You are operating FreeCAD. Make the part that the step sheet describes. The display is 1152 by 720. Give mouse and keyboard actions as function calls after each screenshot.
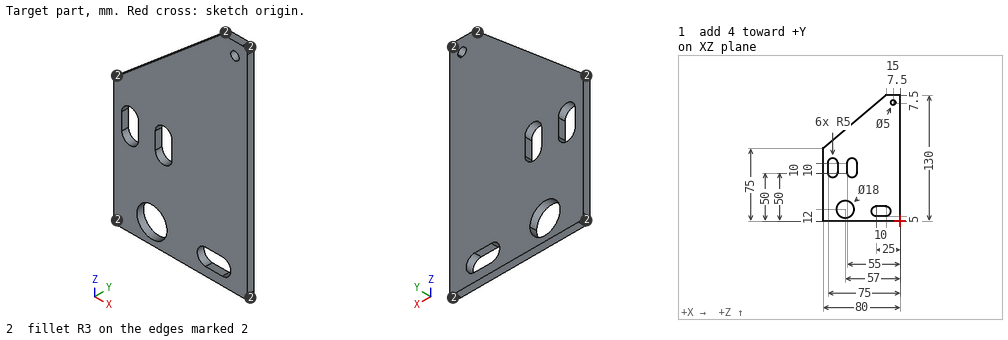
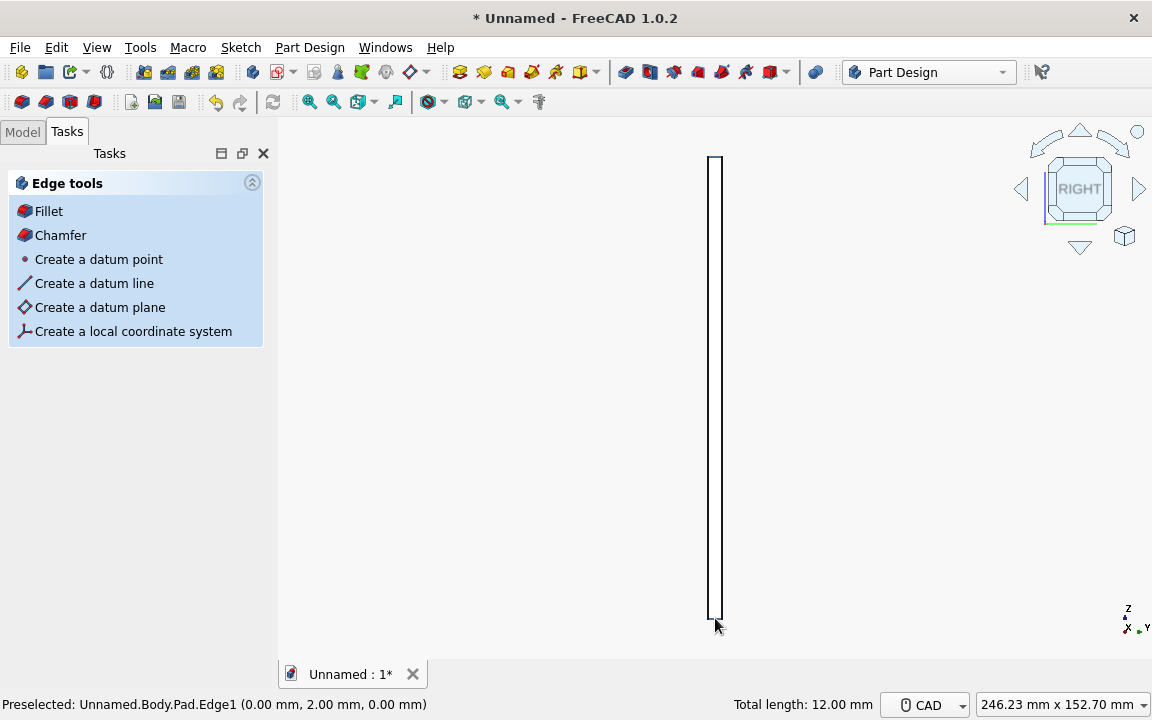
scroll(715, 352, up, 6)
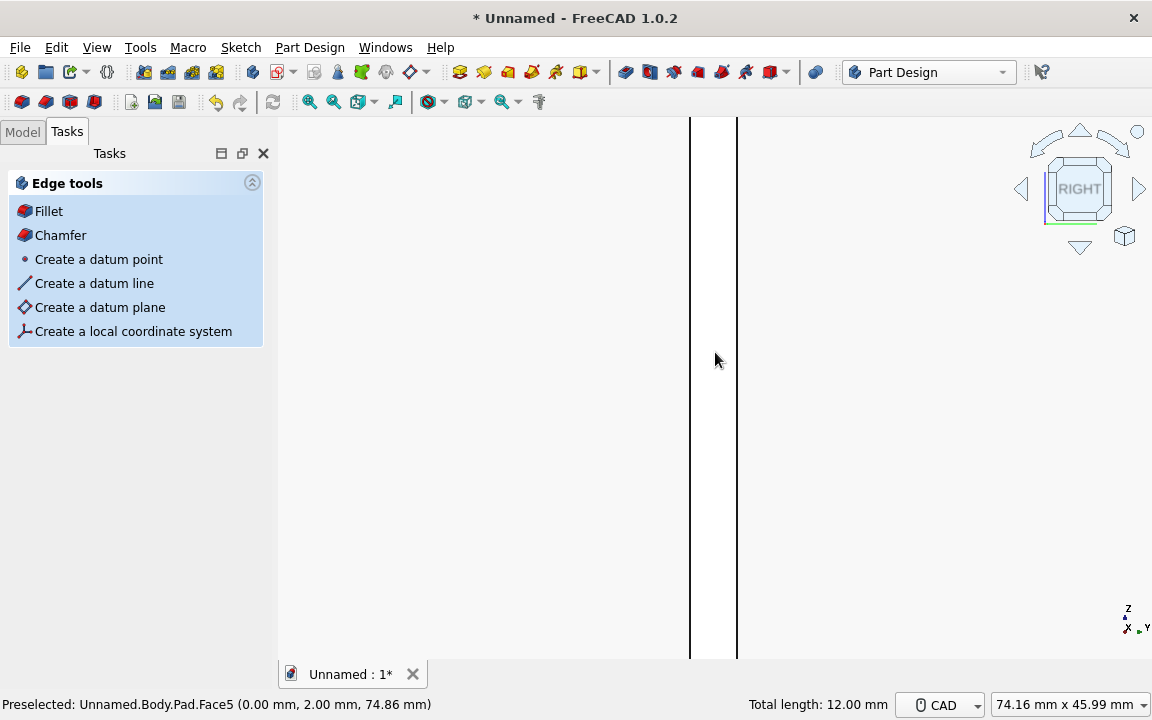
click(310, 102)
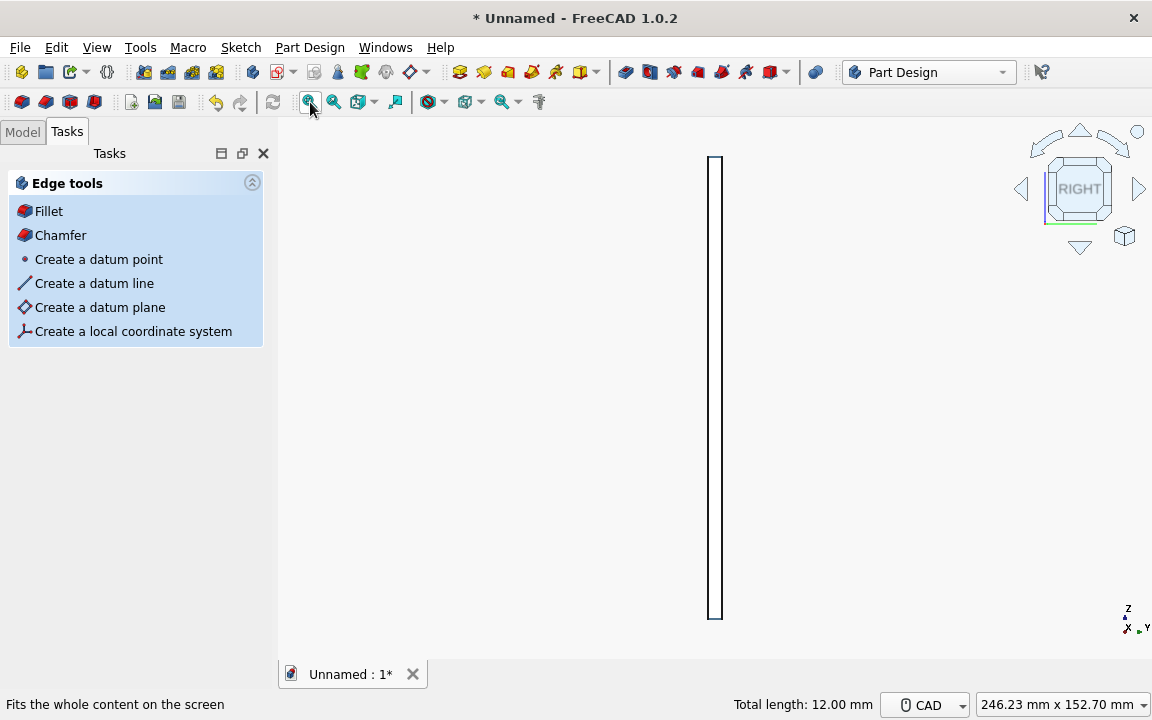
key(5)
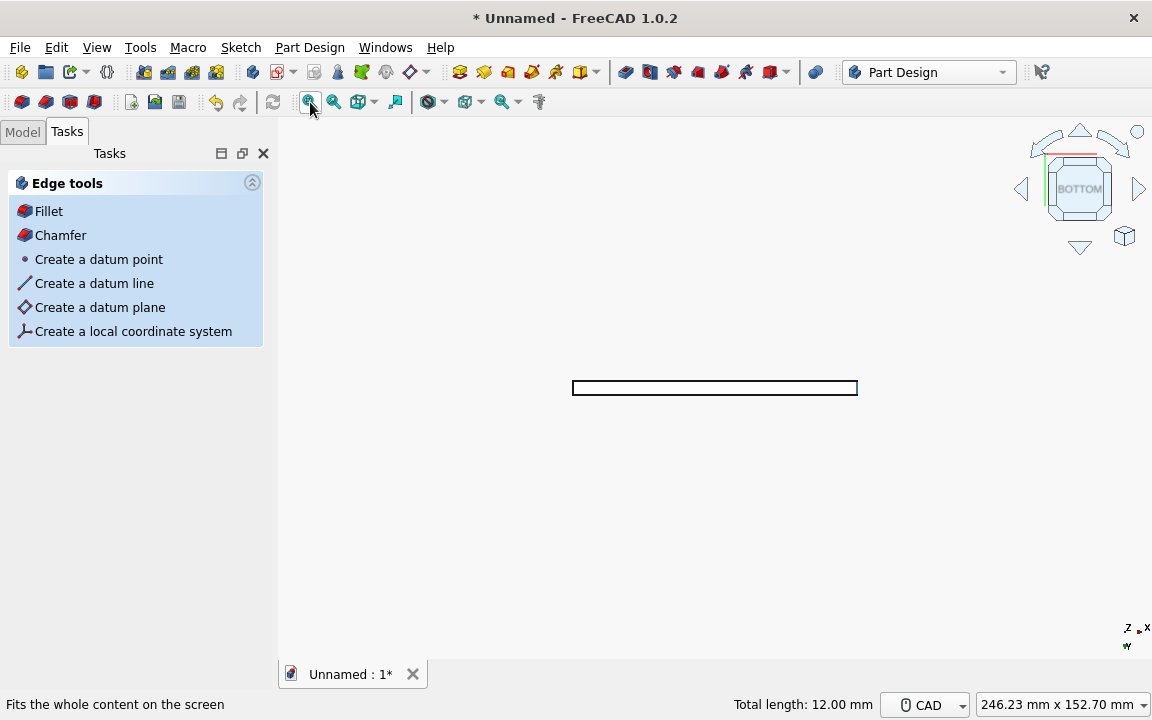
click(310, 102)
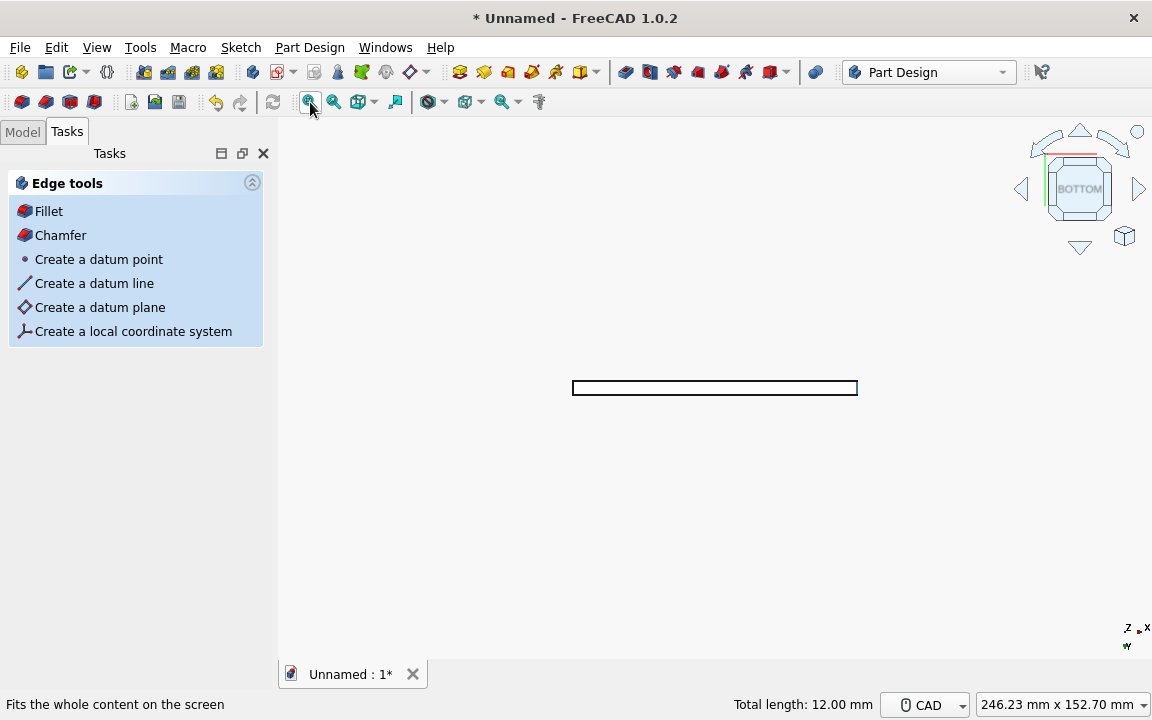
click(573, 387, ctrl)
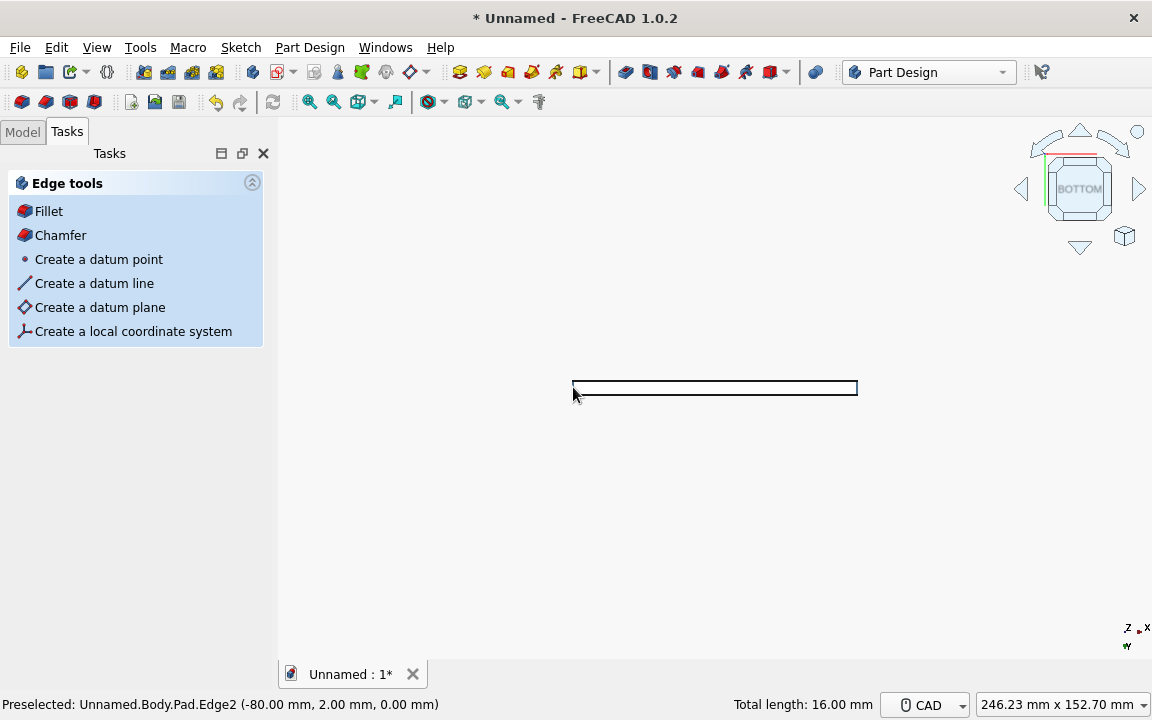
scroll(573, 387, up, 6)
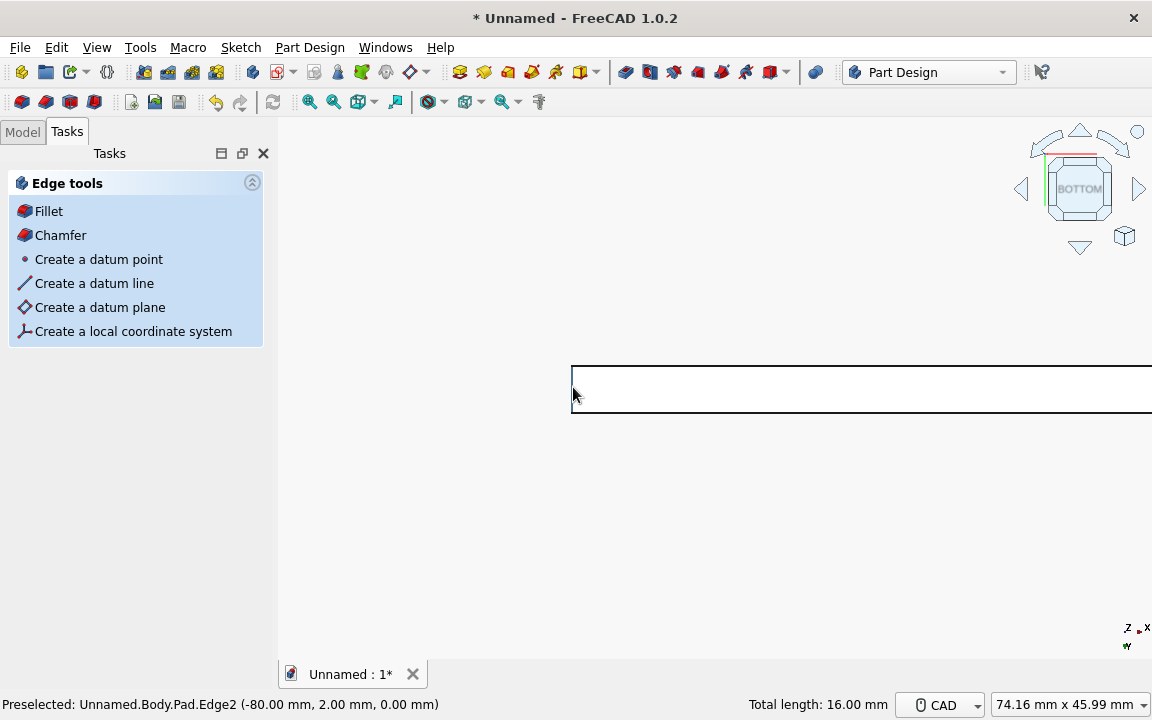
click(310, 102)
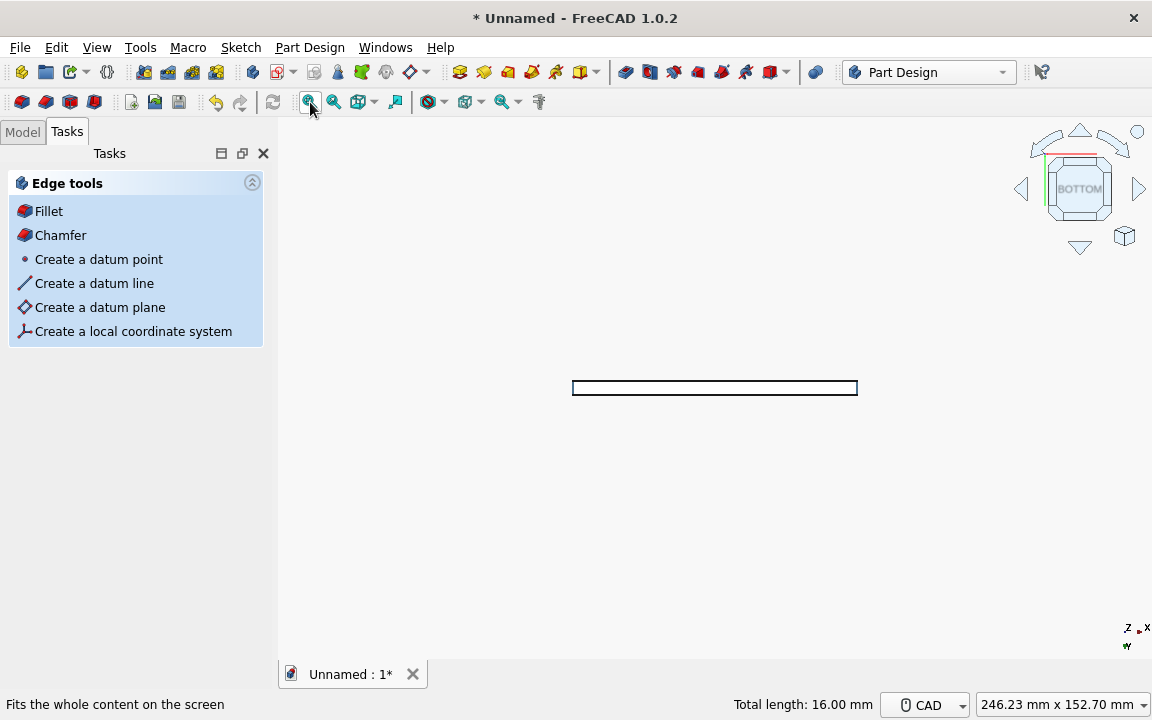
key(4)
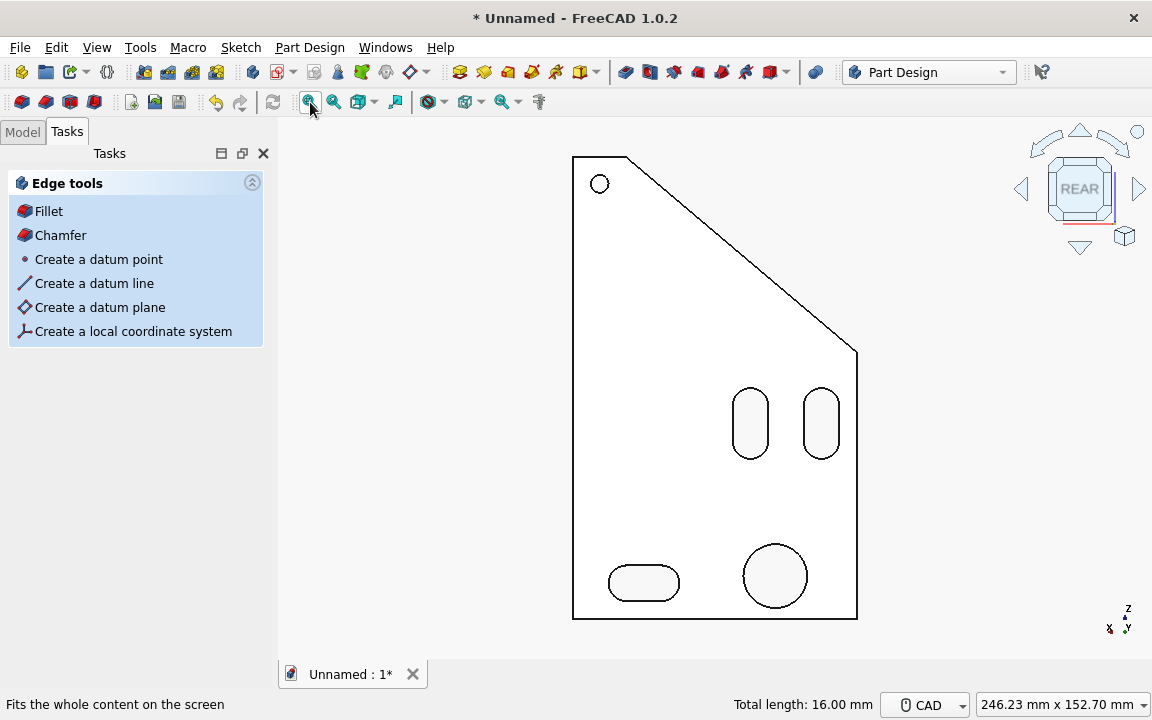
scroll(857, 352, up, 6)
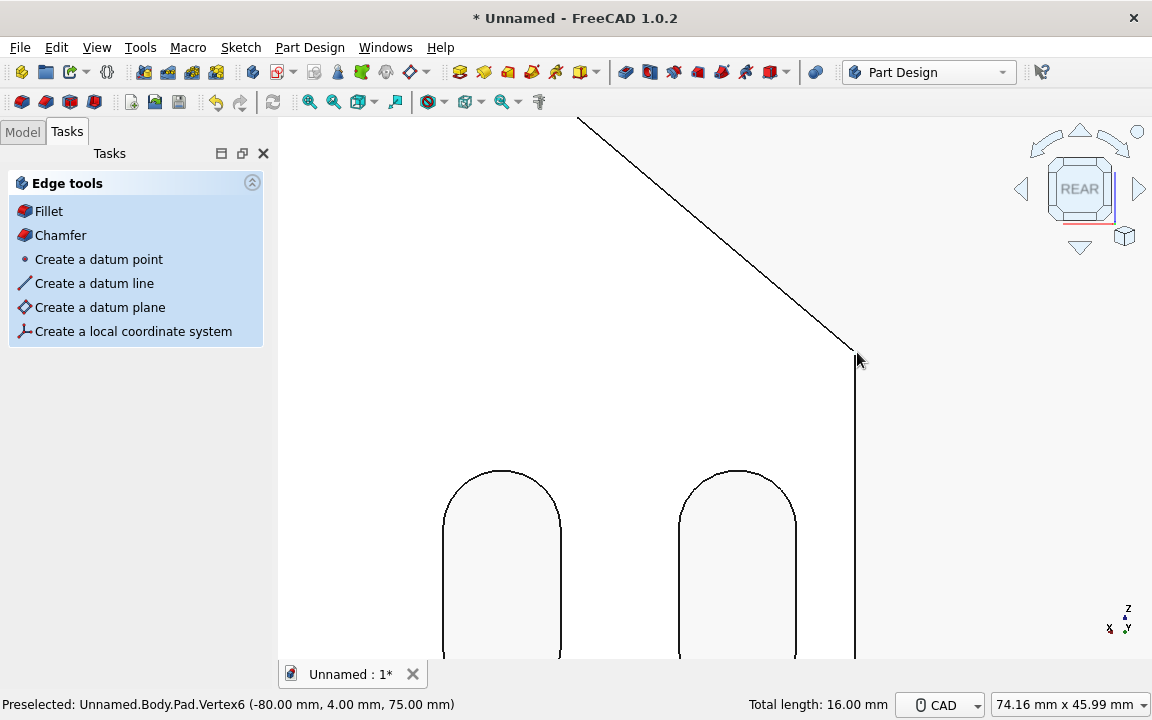
click(310, 102)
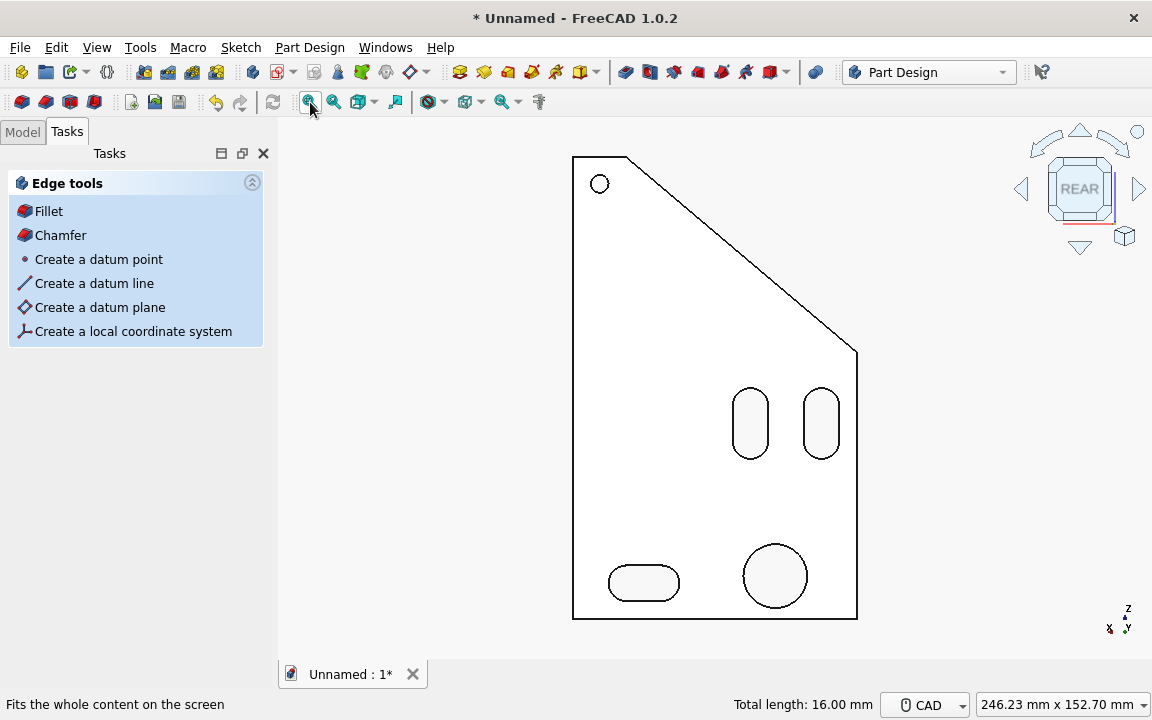
key(6)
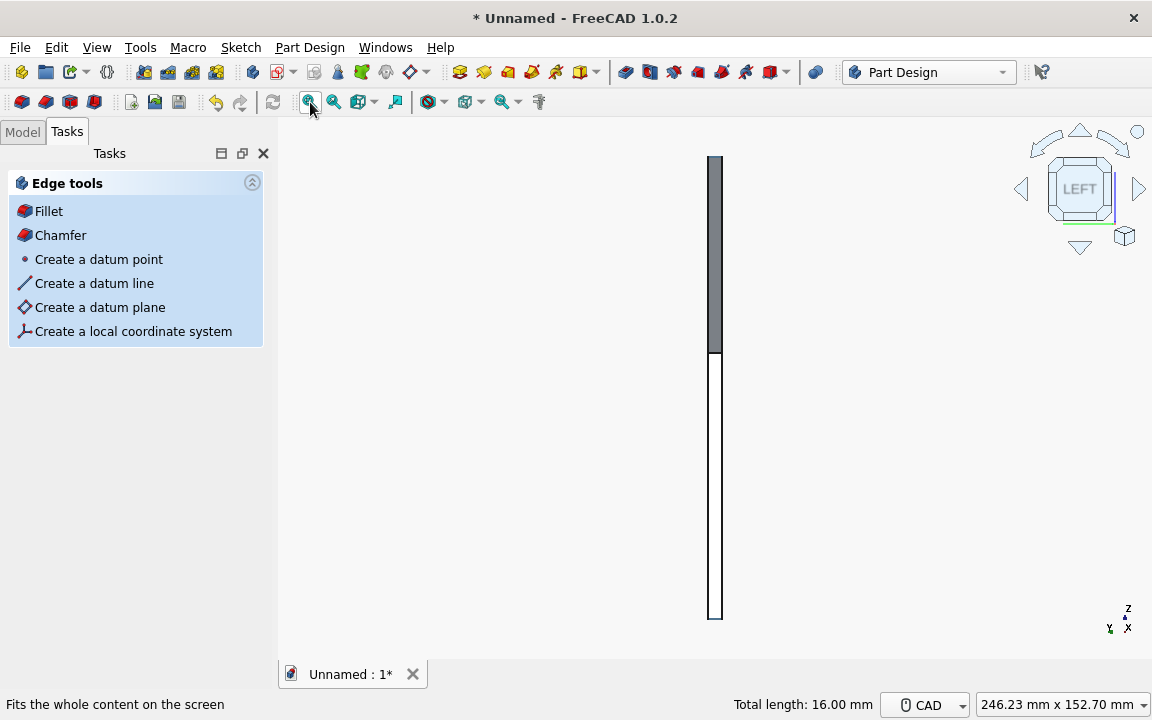
click(715, 352, ctrl)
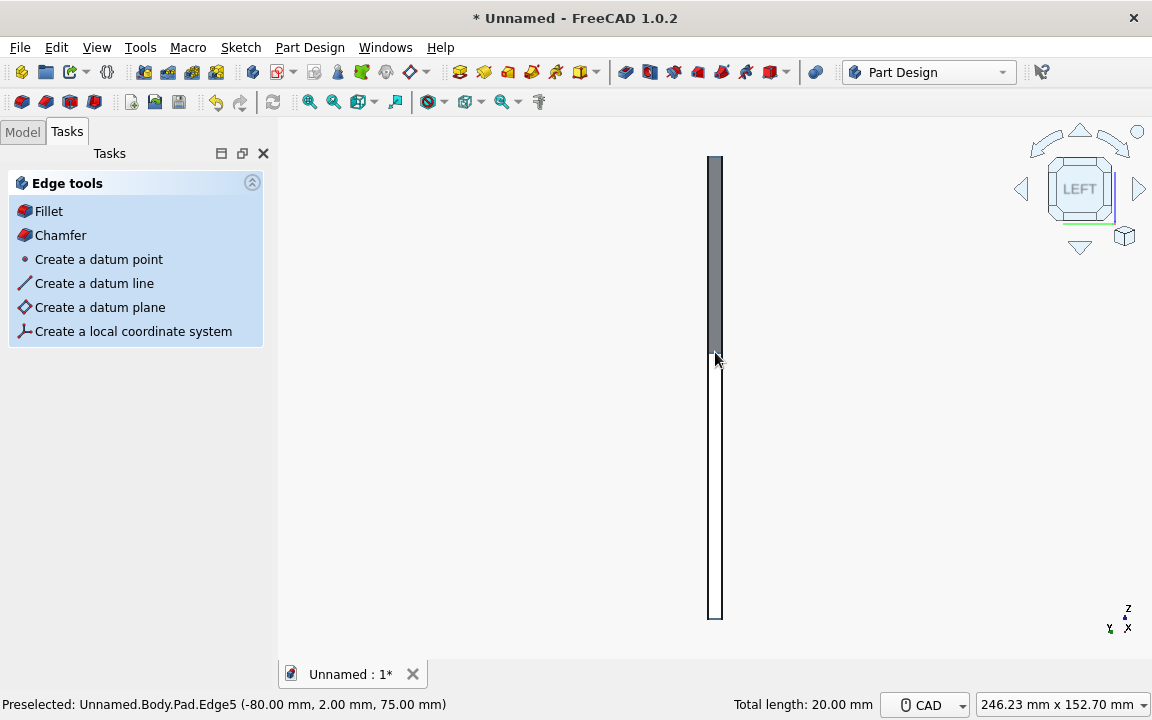
click(22, 102)